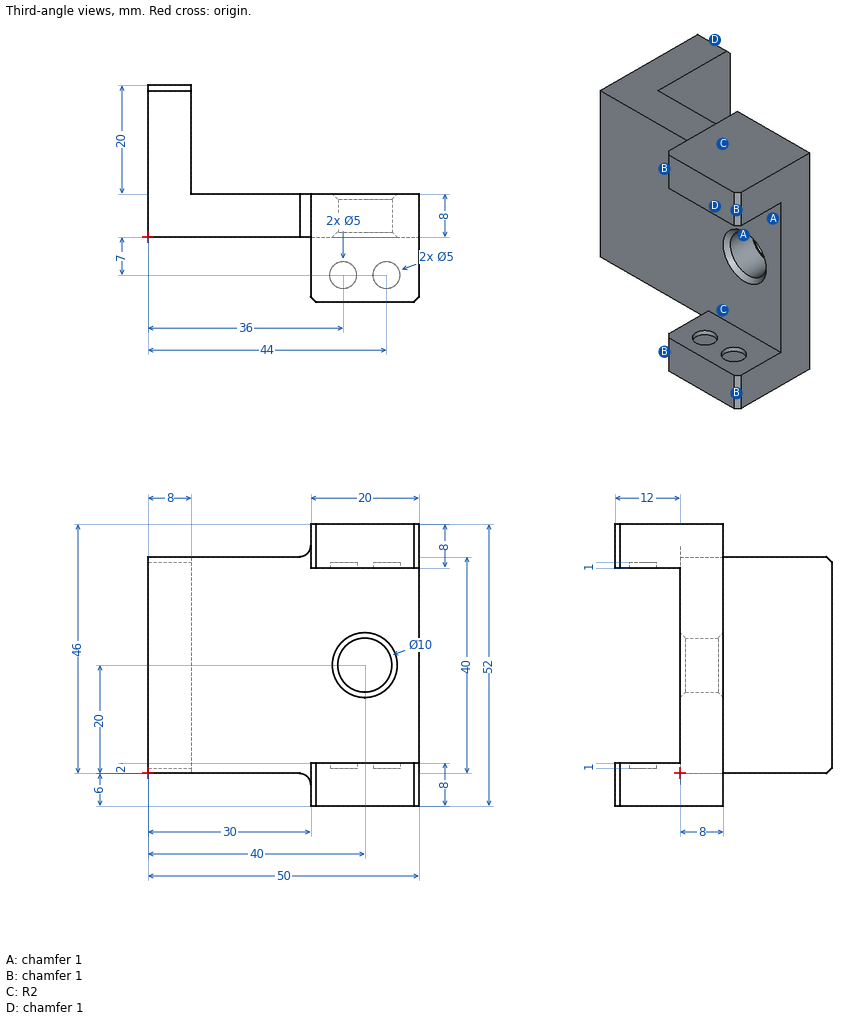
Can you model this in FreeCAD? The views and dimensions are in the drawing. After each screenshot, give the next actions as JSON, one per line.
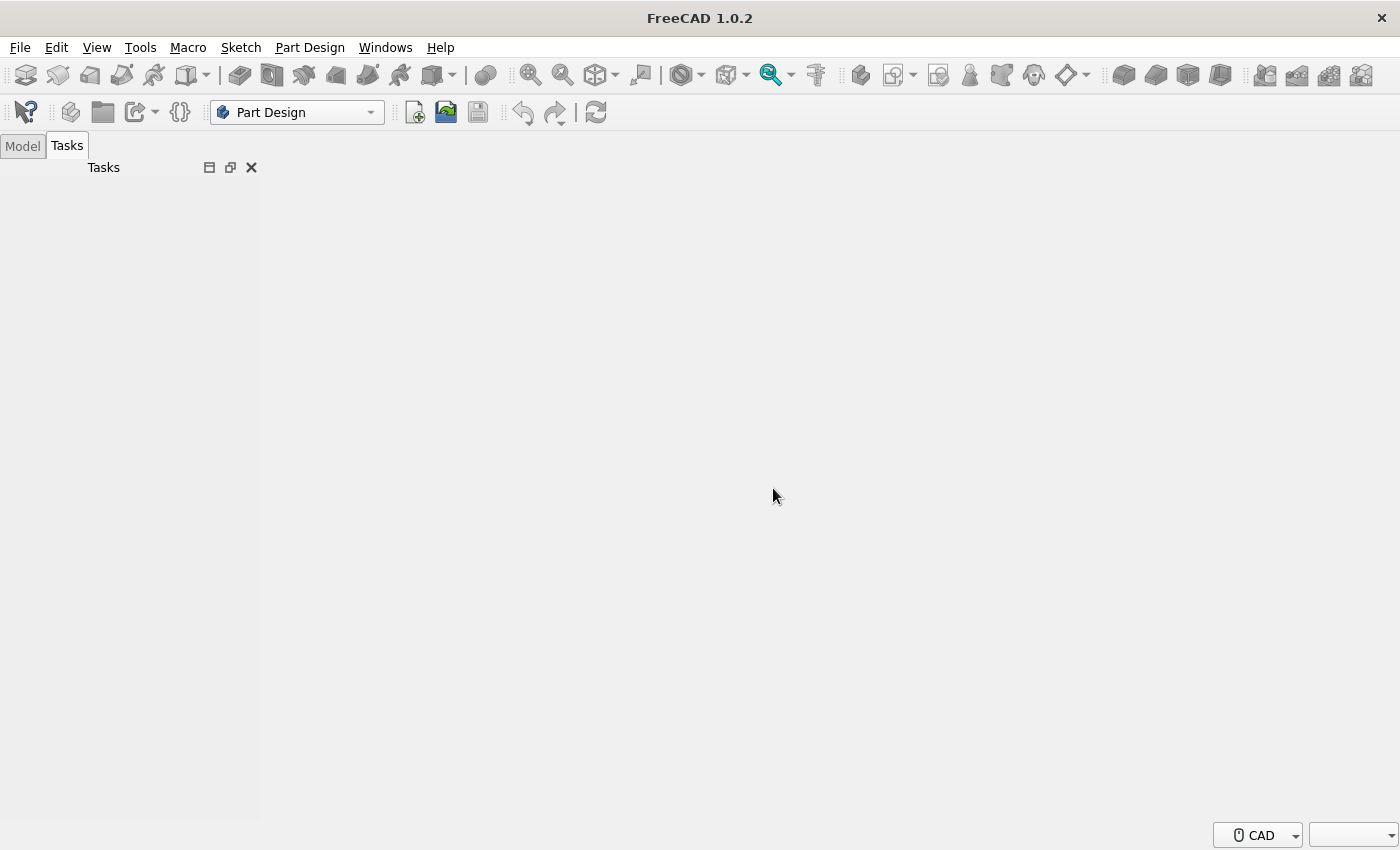
{"action": "left_click", "coordinate": [414, 112]}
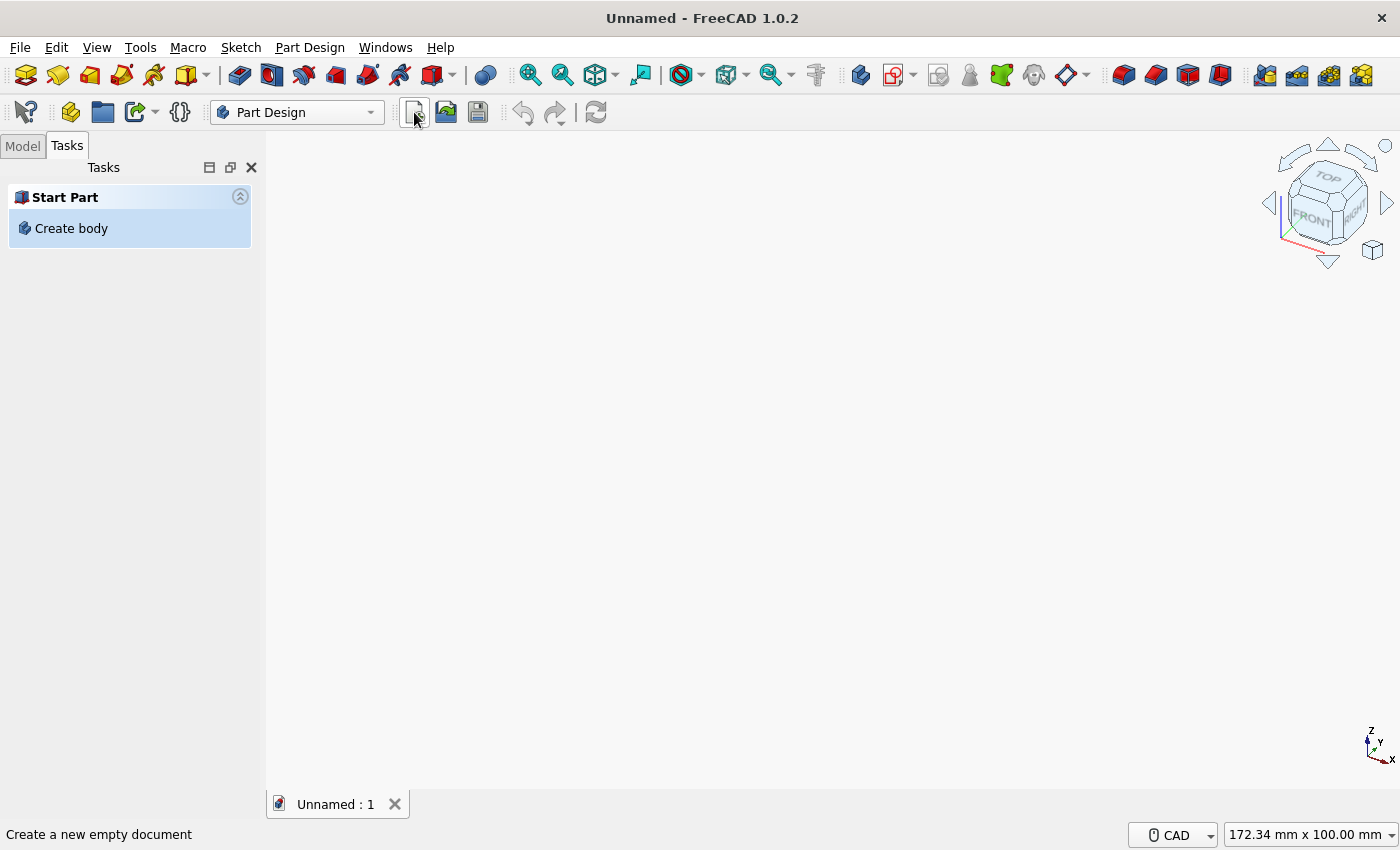
{"action": "left_click", "coordinate": [894, 76]}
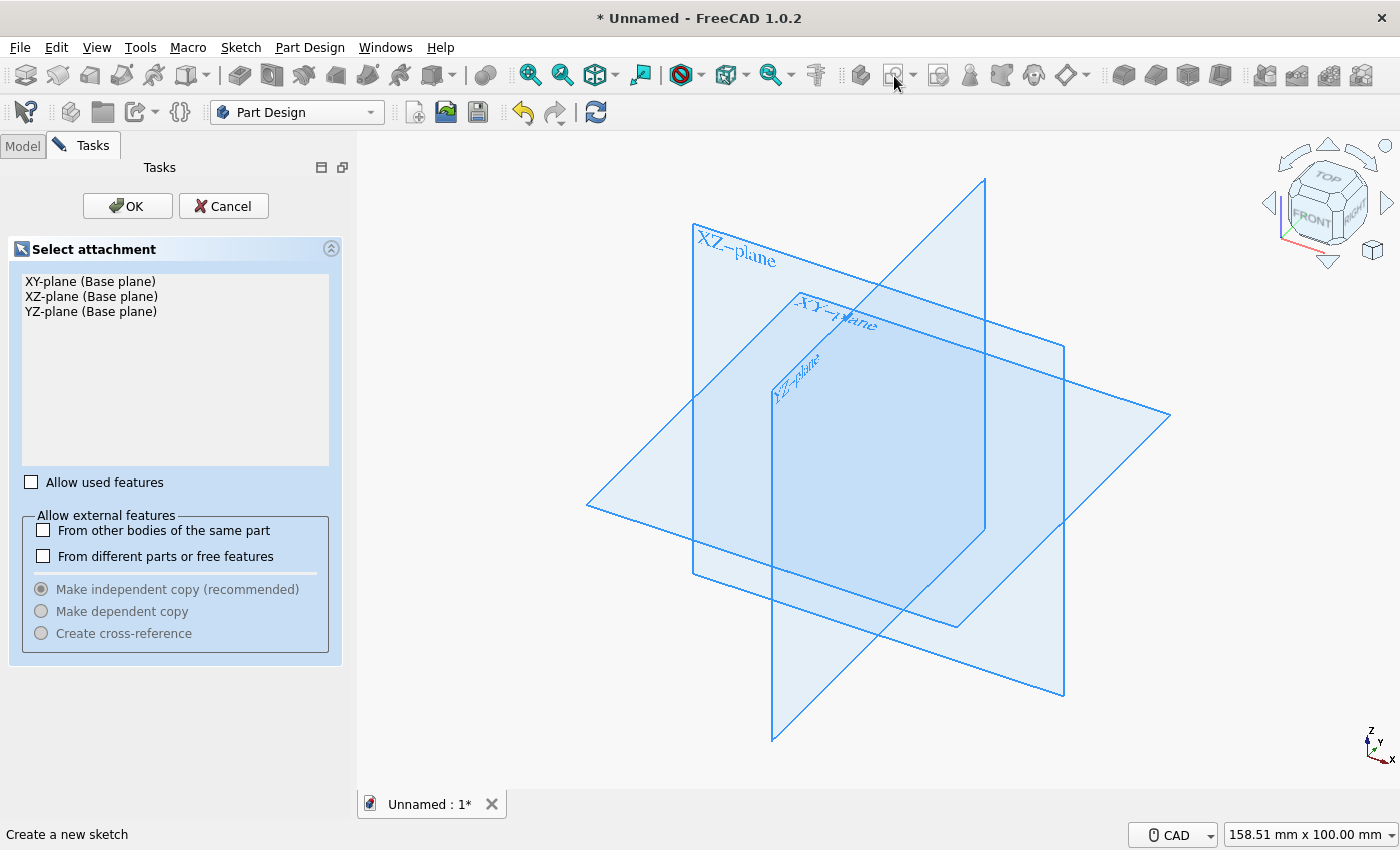
{"action": "left_click", "coordinate": [82, 296]}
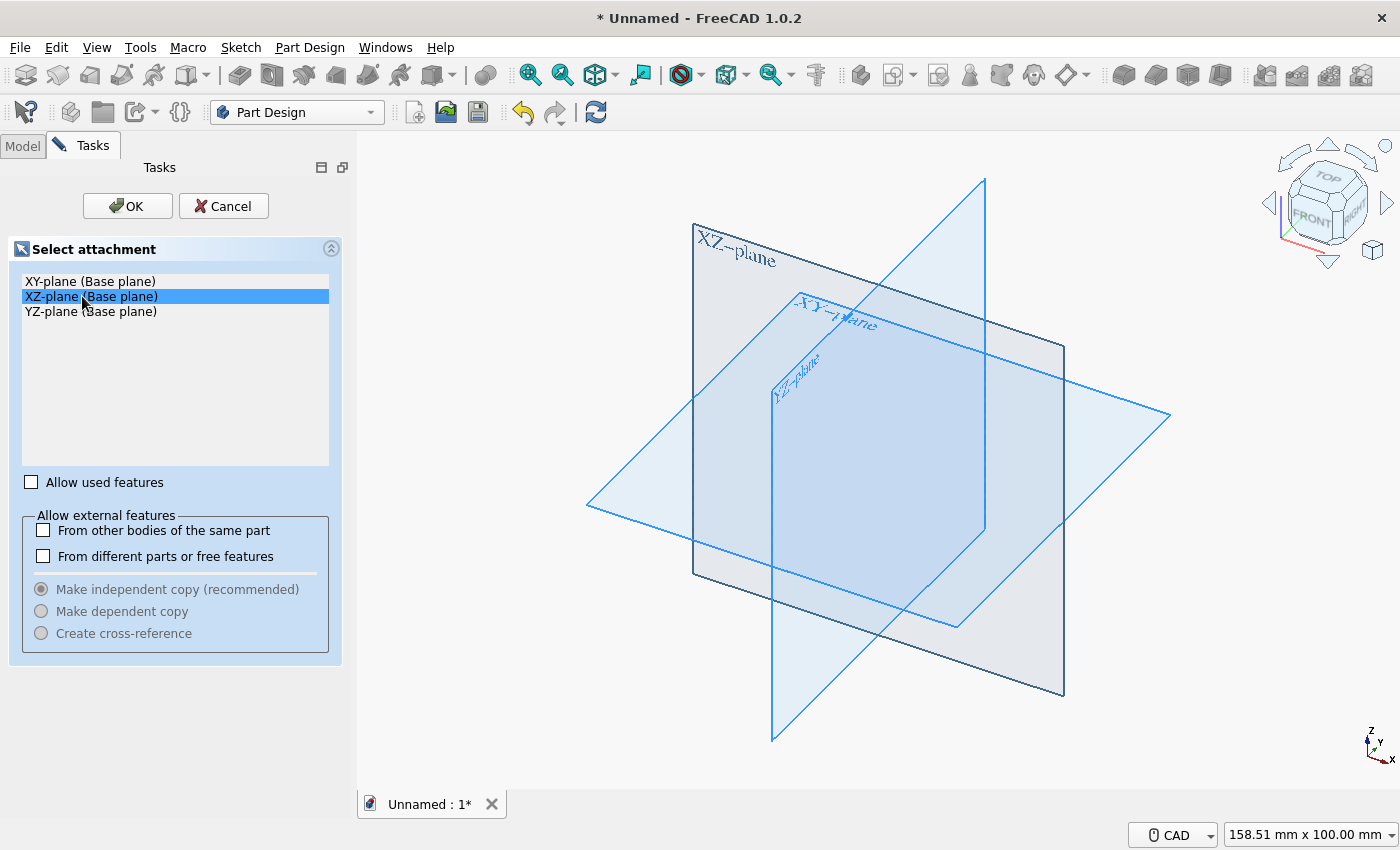
{"action": "left_click", "coordinate": [128, 206]}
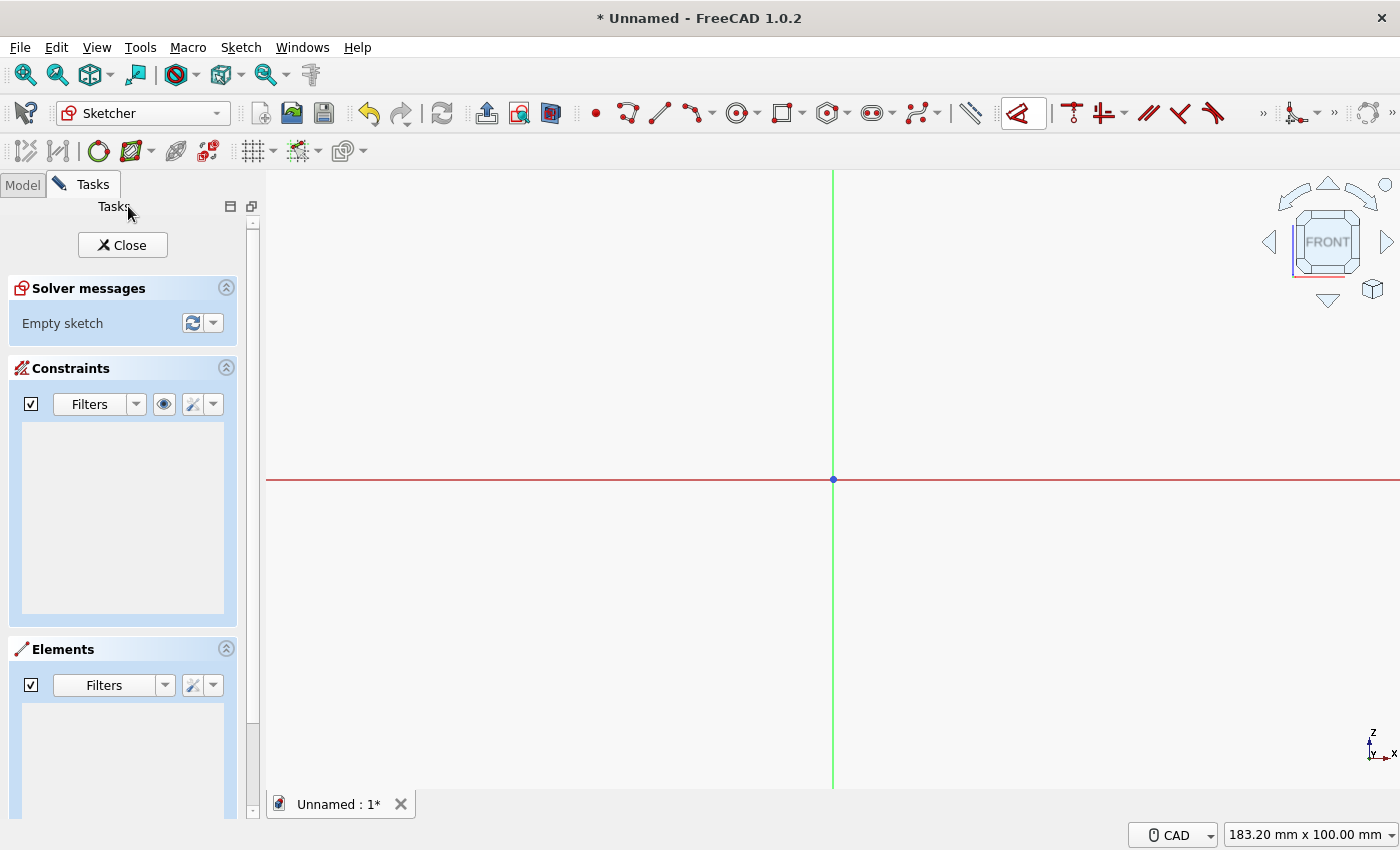
{"action": "scroll", "coordinate": [1235, 198], "scroll_direction": "up", "scroll_amount": 2}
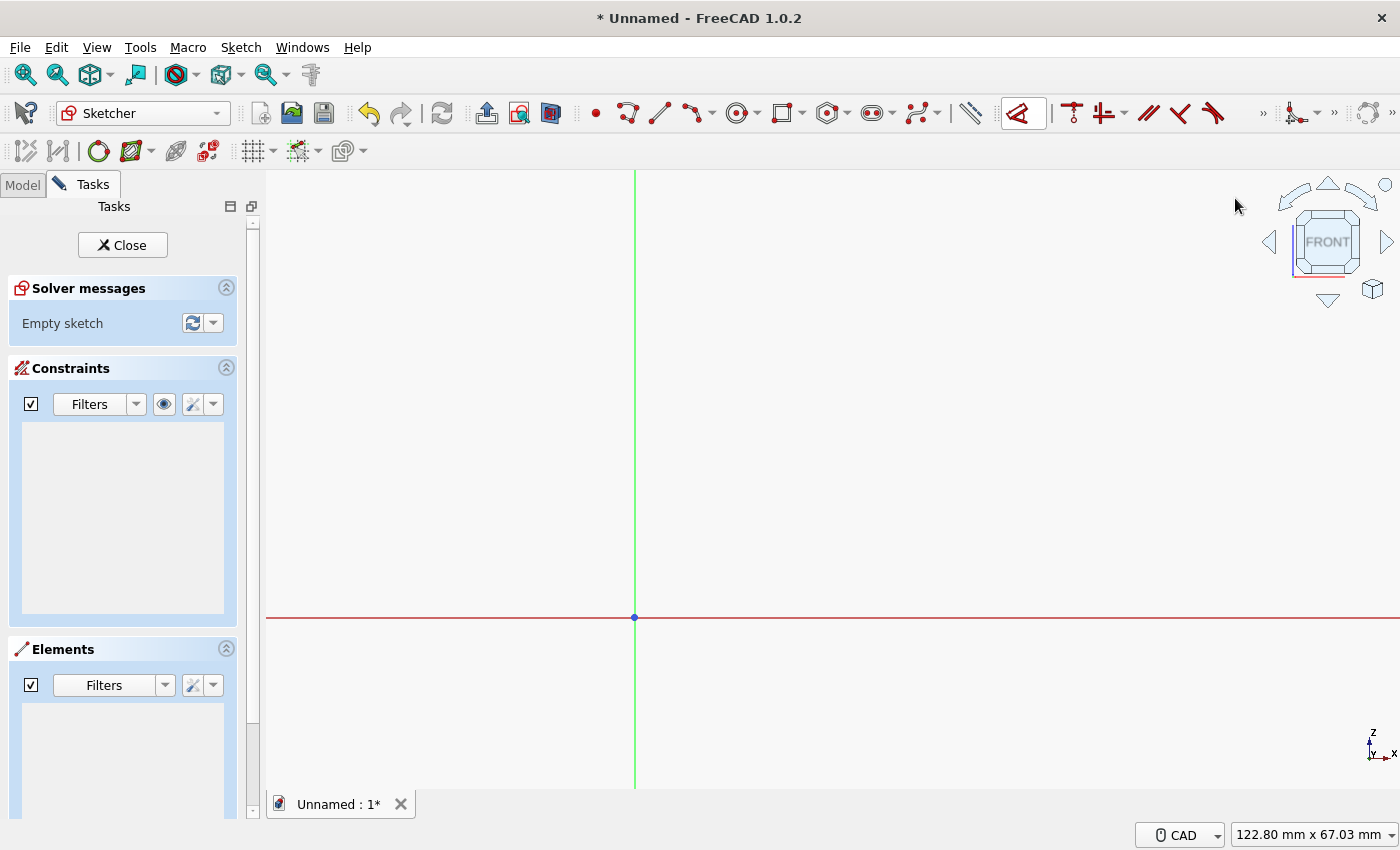
{"action": "left_click", "coordinate": [782, 114]}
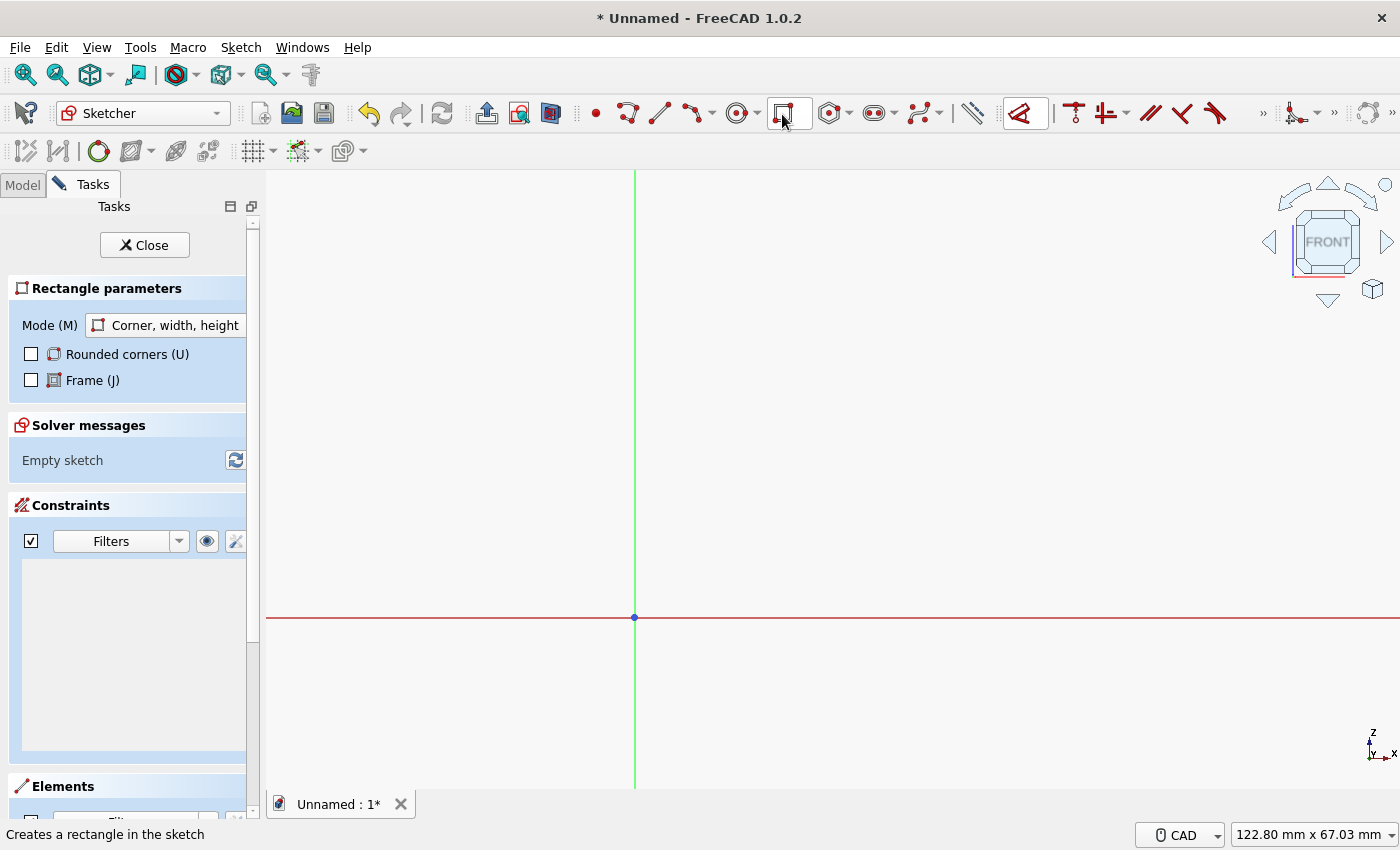
{"action": "left_click", "coordinate": [635, 618]}
{"action": "mouse_move", "coordinate": [1097, 249]}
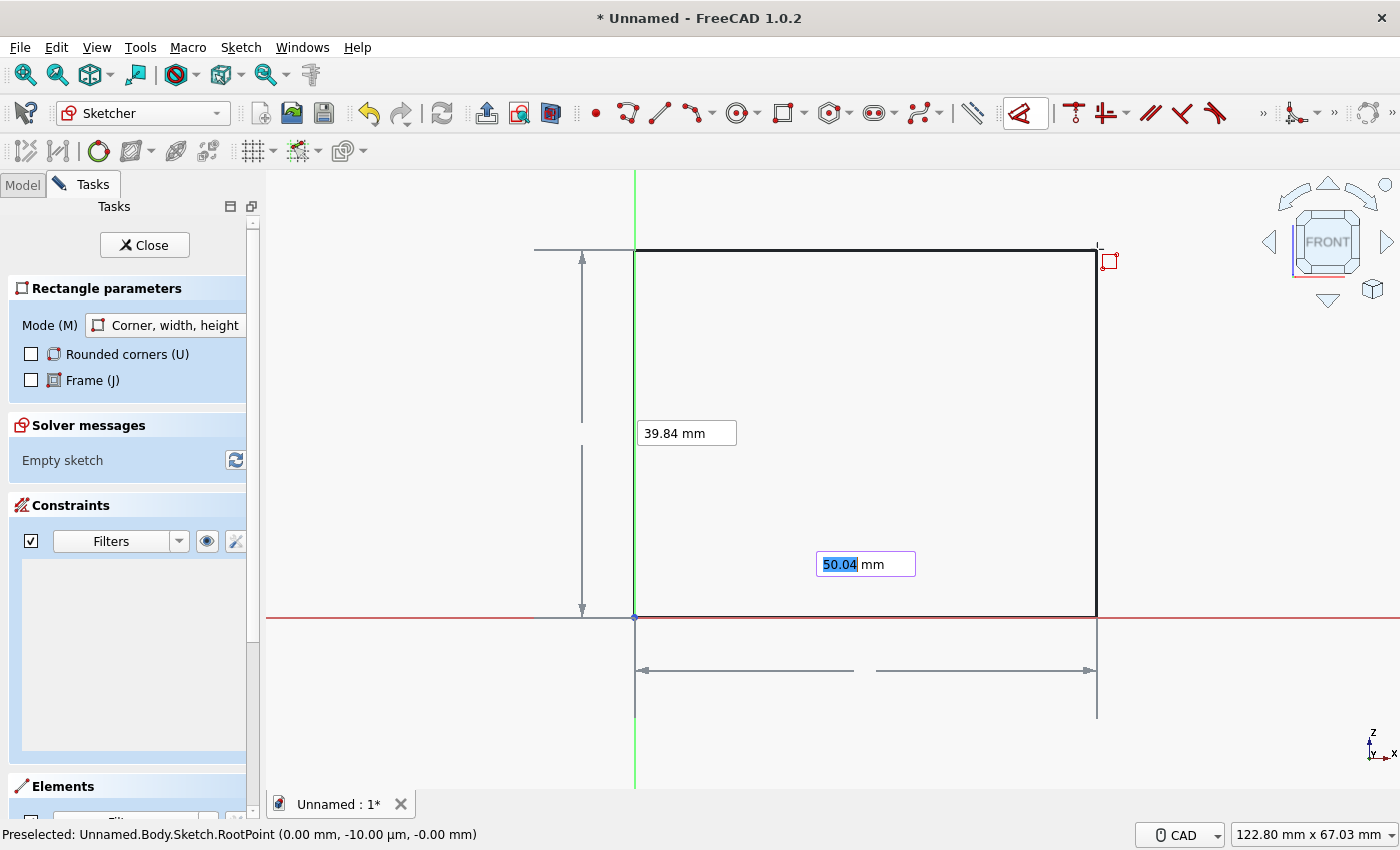
{"action": "type", "text": "50"}
{"action": "key", "text": "Tab"}
{"action": "type", "text": "40"}
{"action": "key", "text": "Return"}
{"action": "key", "text": "Escape"}